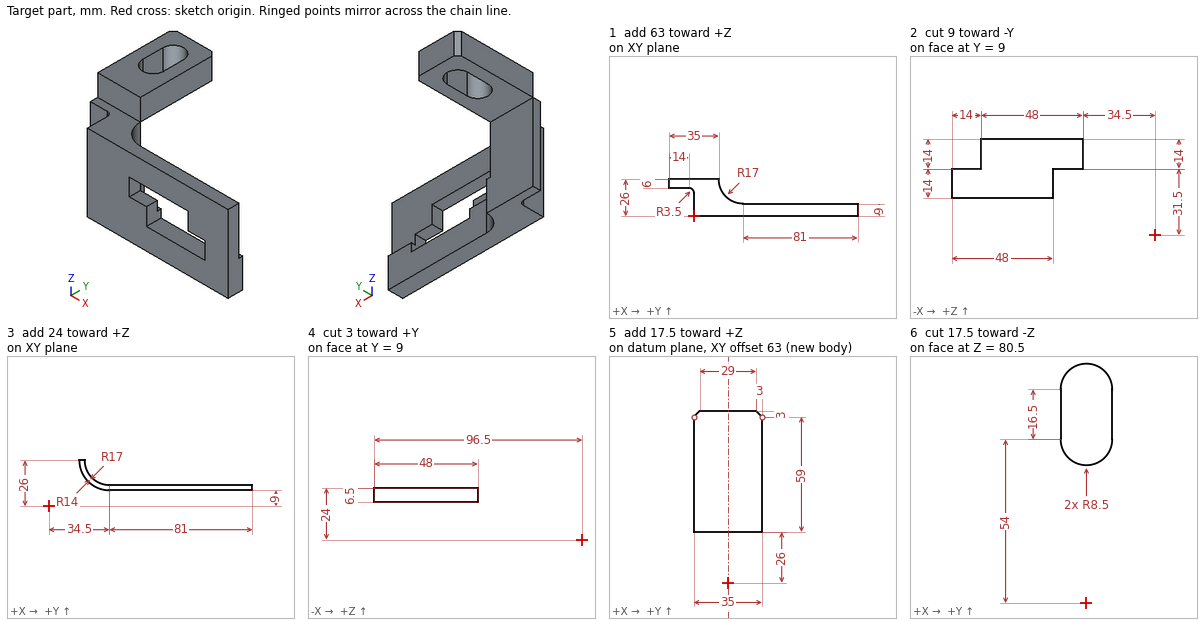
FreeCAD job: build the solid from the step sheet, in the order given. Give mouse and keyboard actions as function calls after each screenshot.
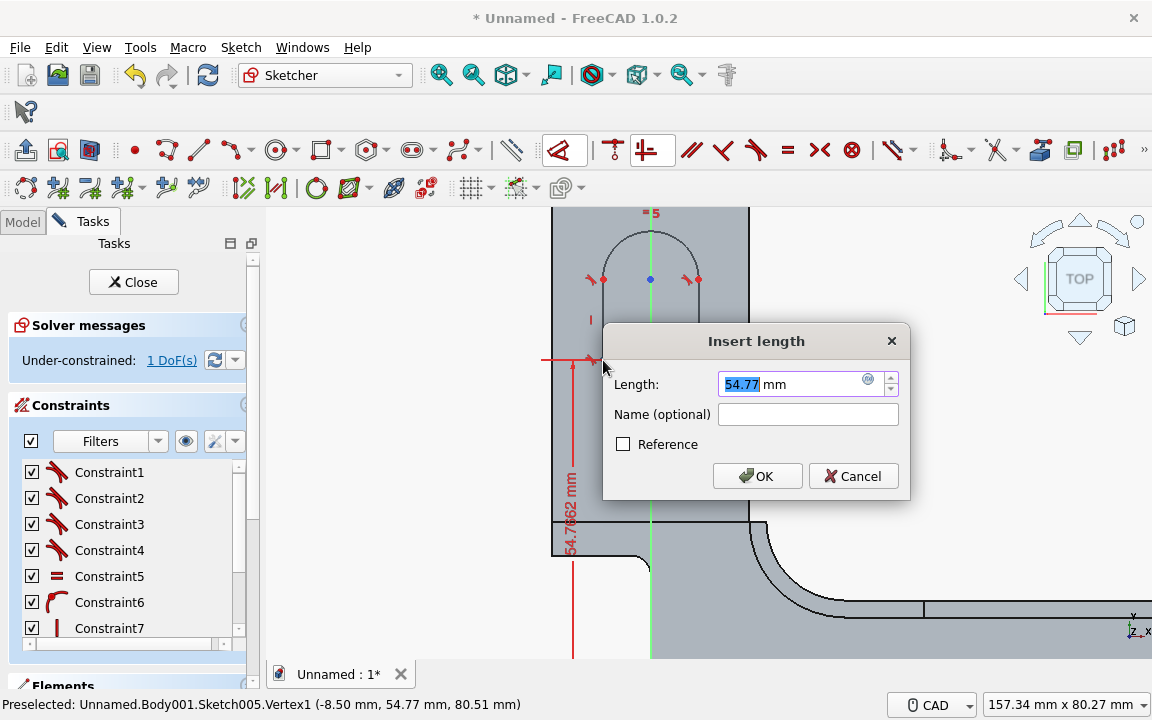
text(54)
key(Return)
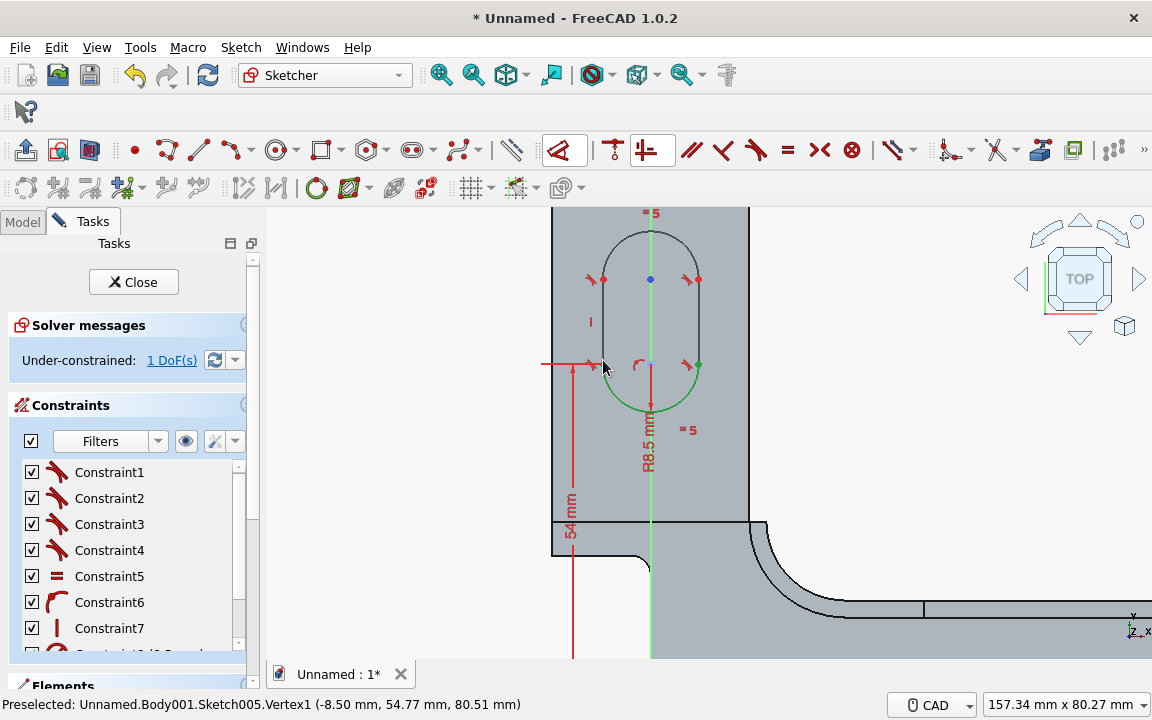
click(603, 339)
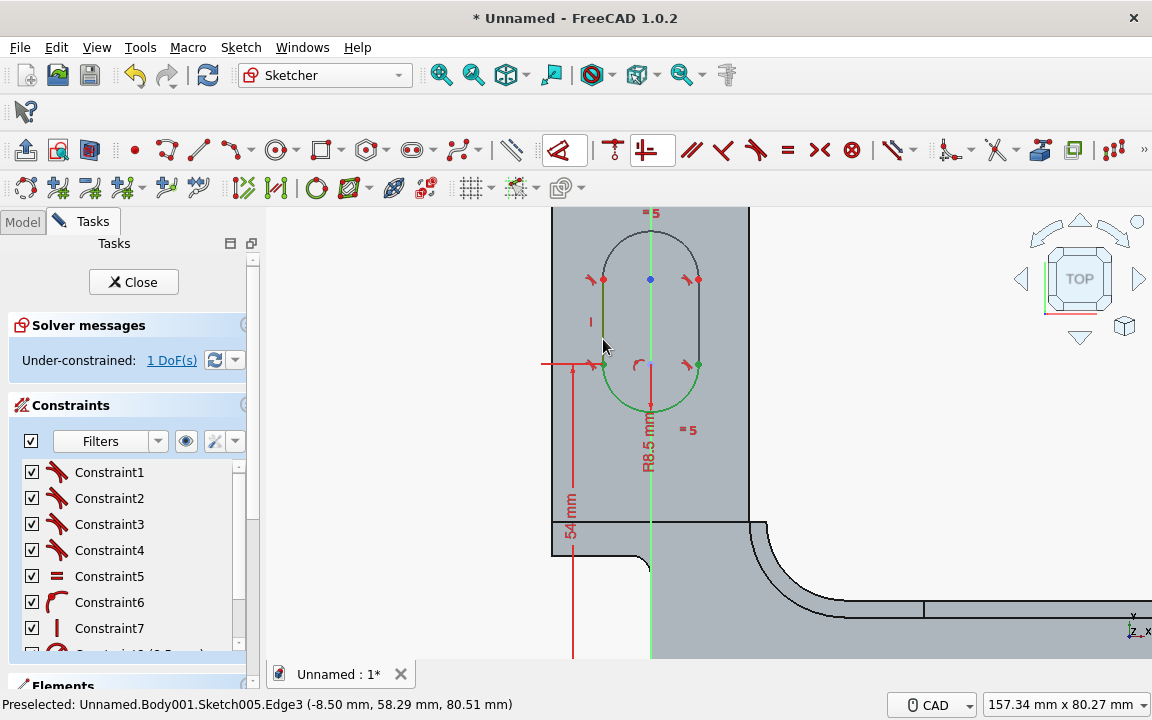
key(i)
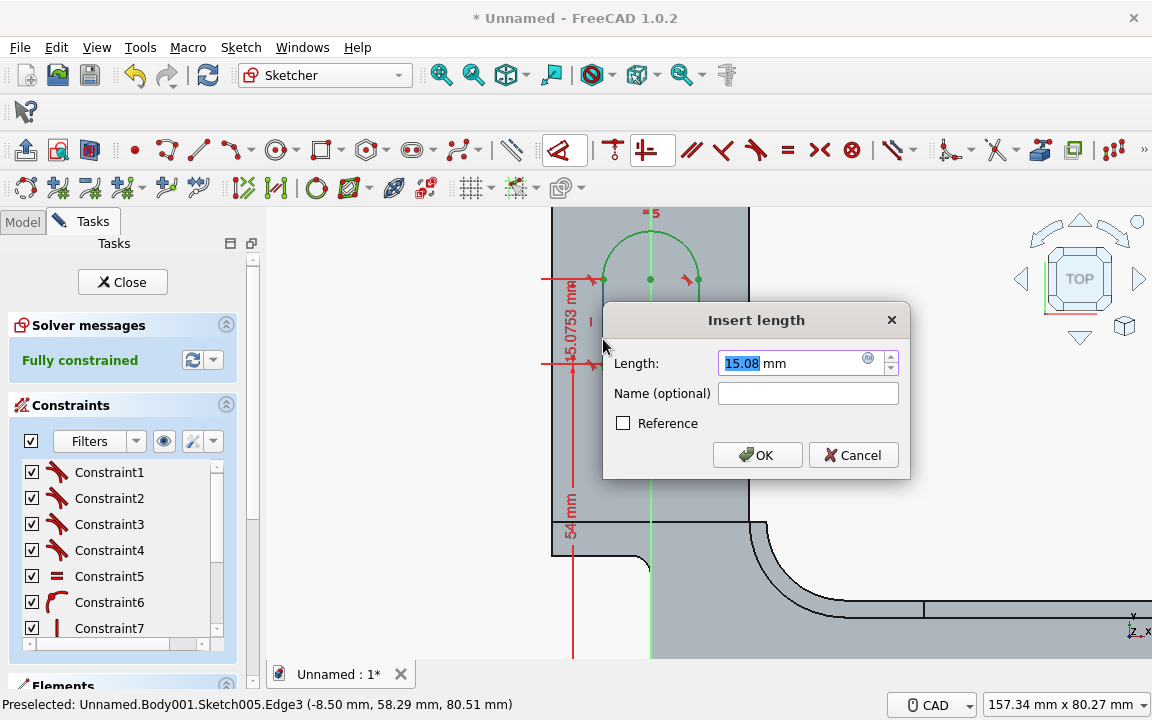
text(16.5)
key(Return)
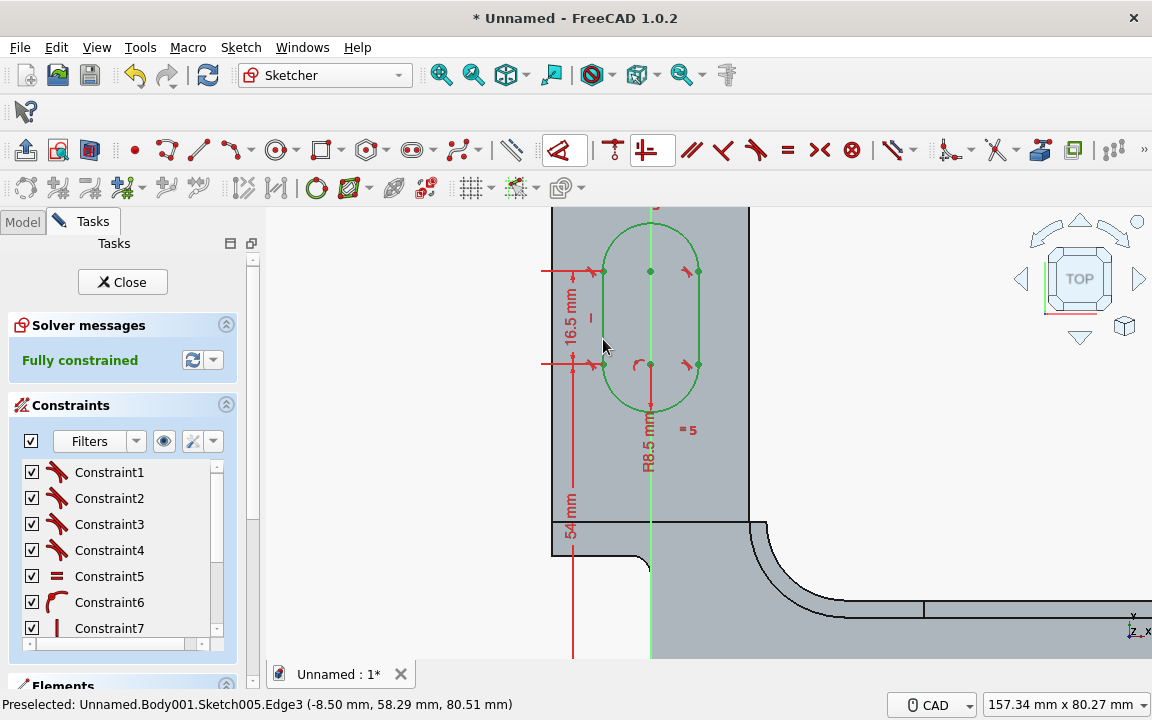
click(123, 282)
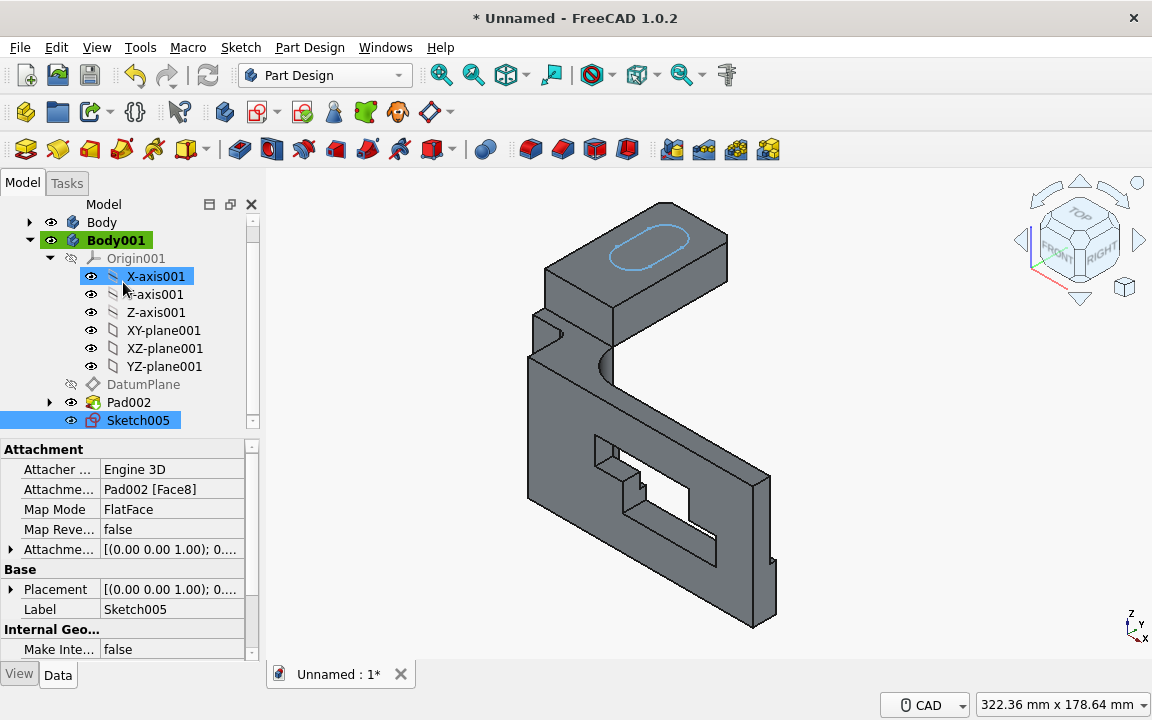
click(240, 150)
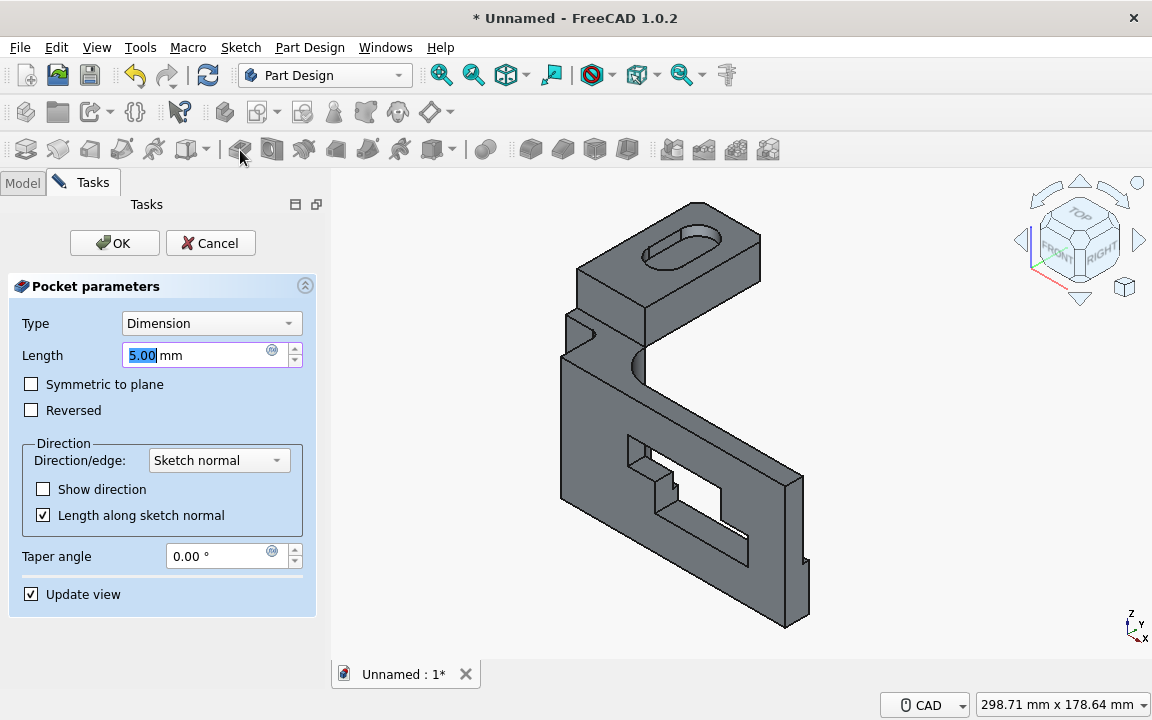
text(17.5)
key(Tab)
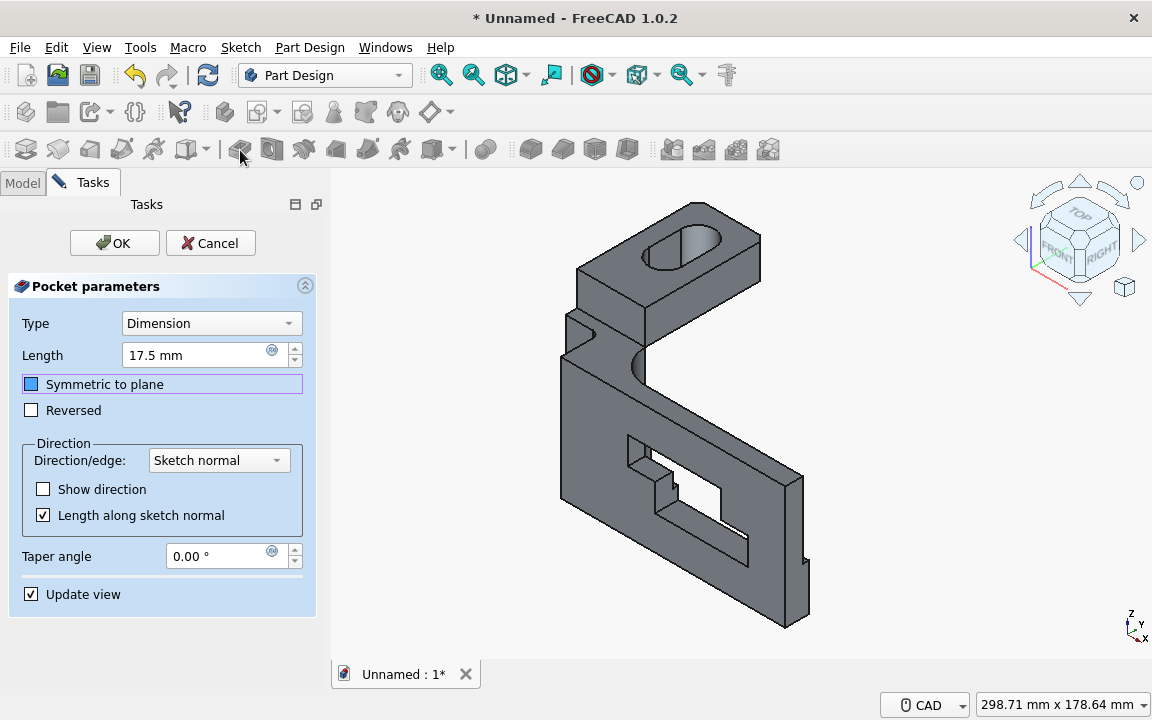
click(115, 243)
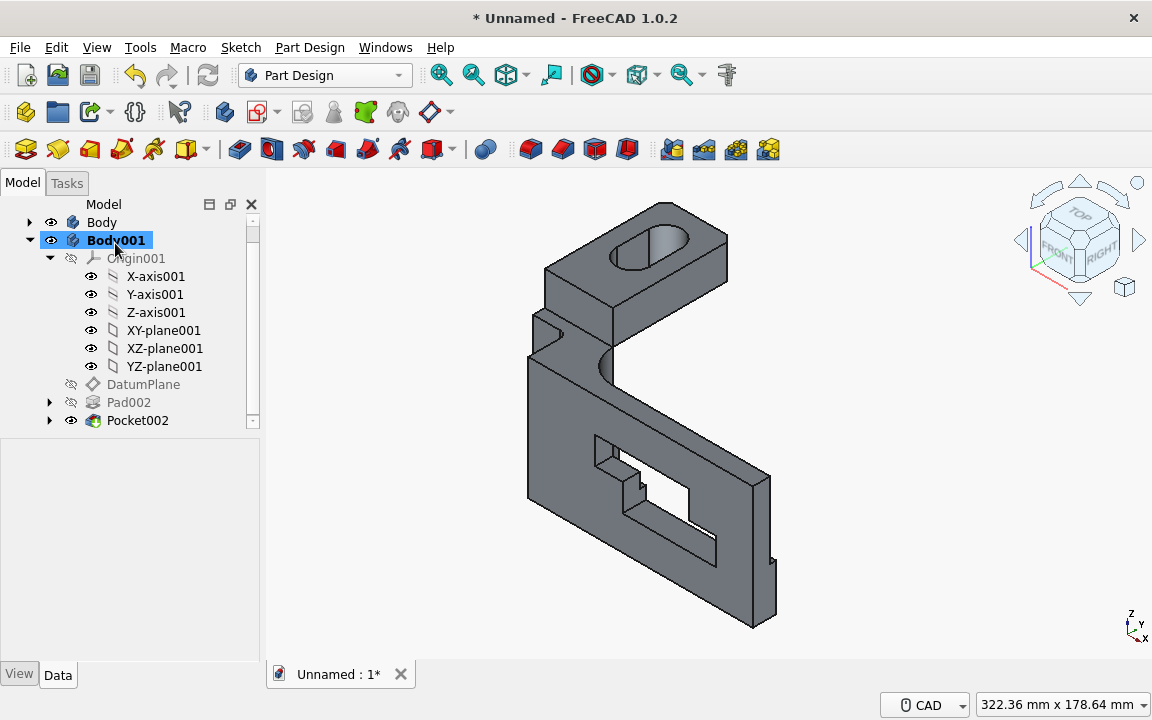
click(442, 76)